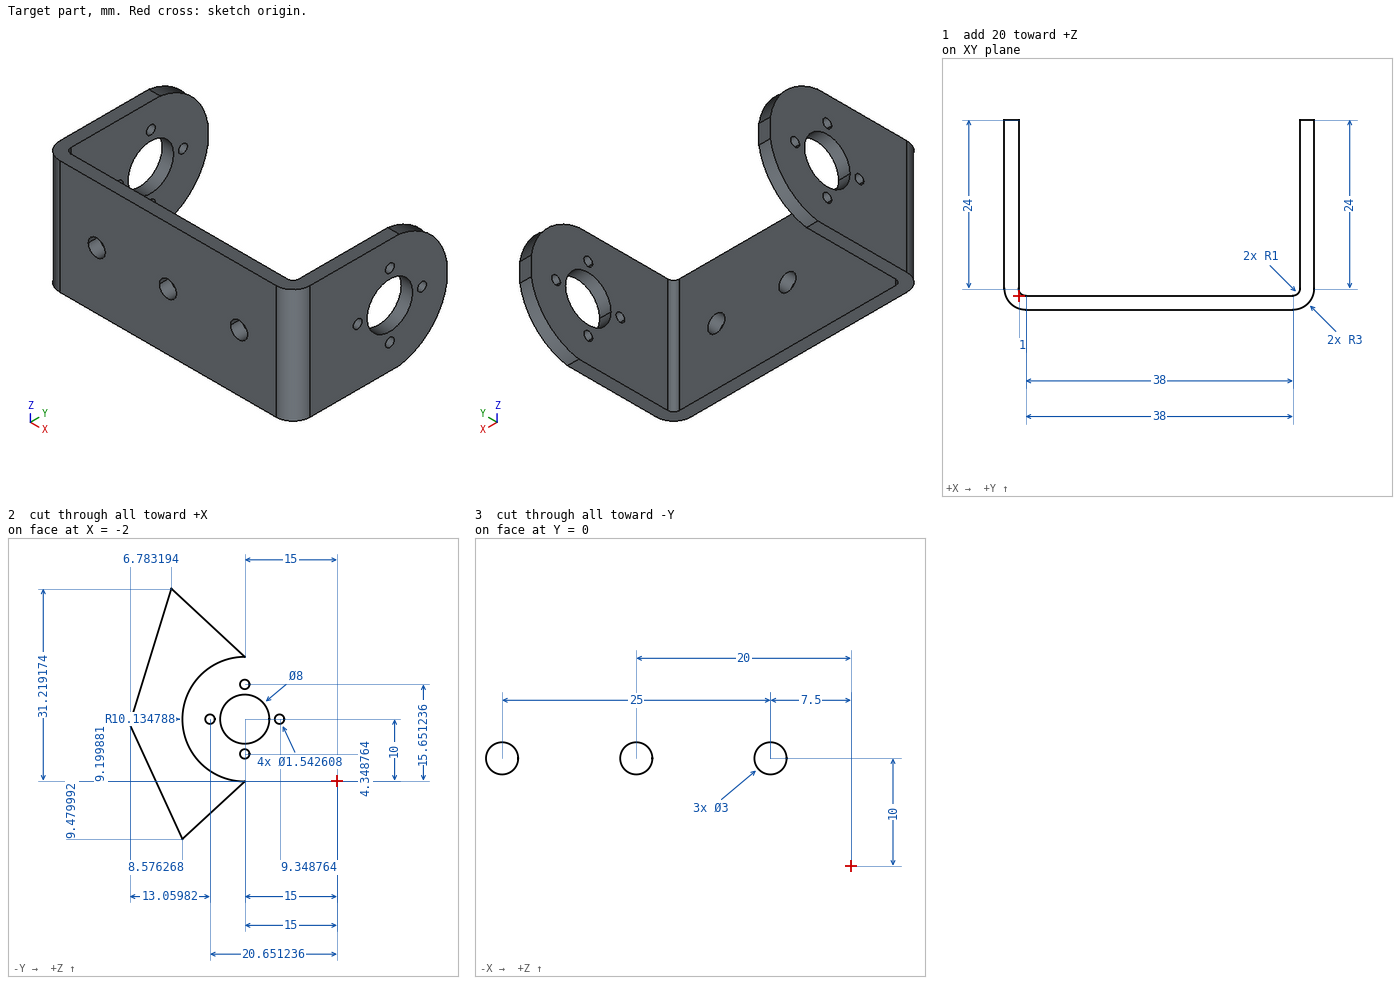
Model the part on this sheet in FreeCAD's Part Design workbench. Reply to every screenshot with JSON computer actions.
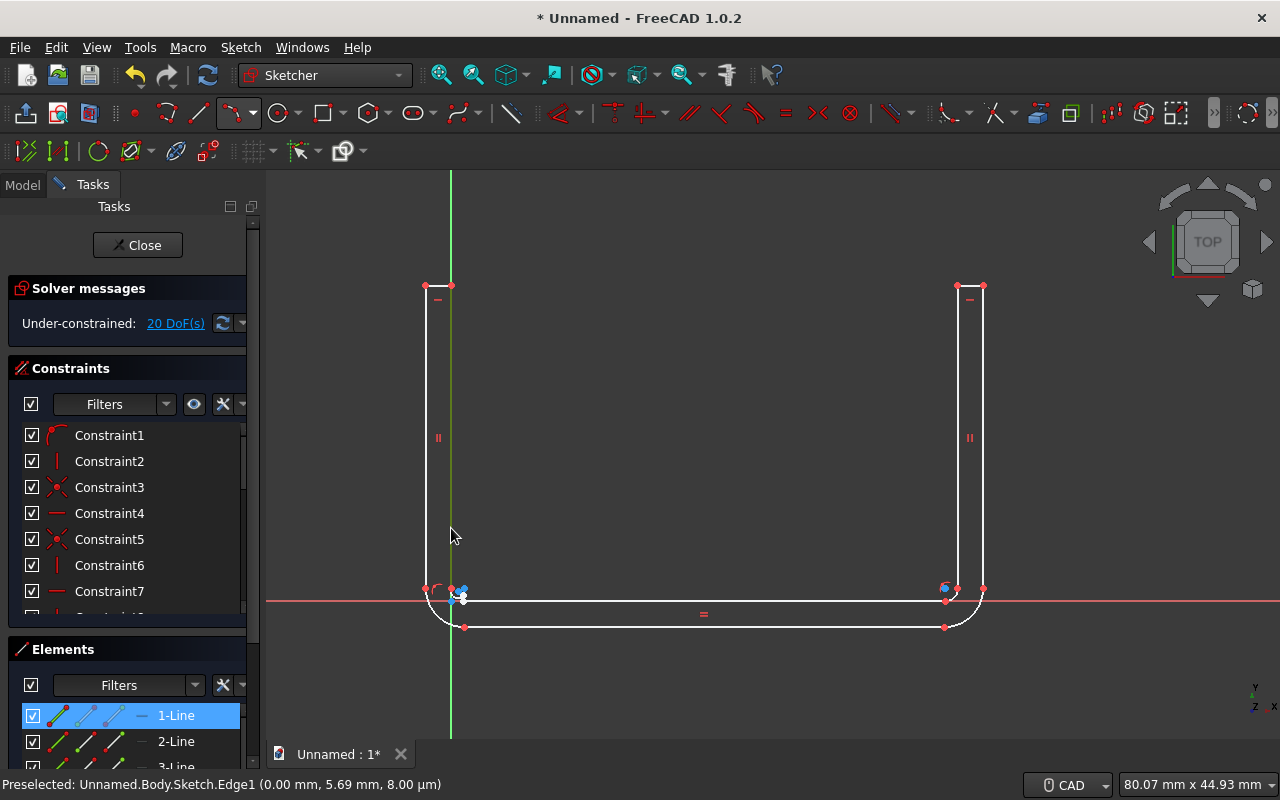
{"action": "scroll", "coordinate": [455, 597], "scroll_direction": "up", "scroll_amount": 4}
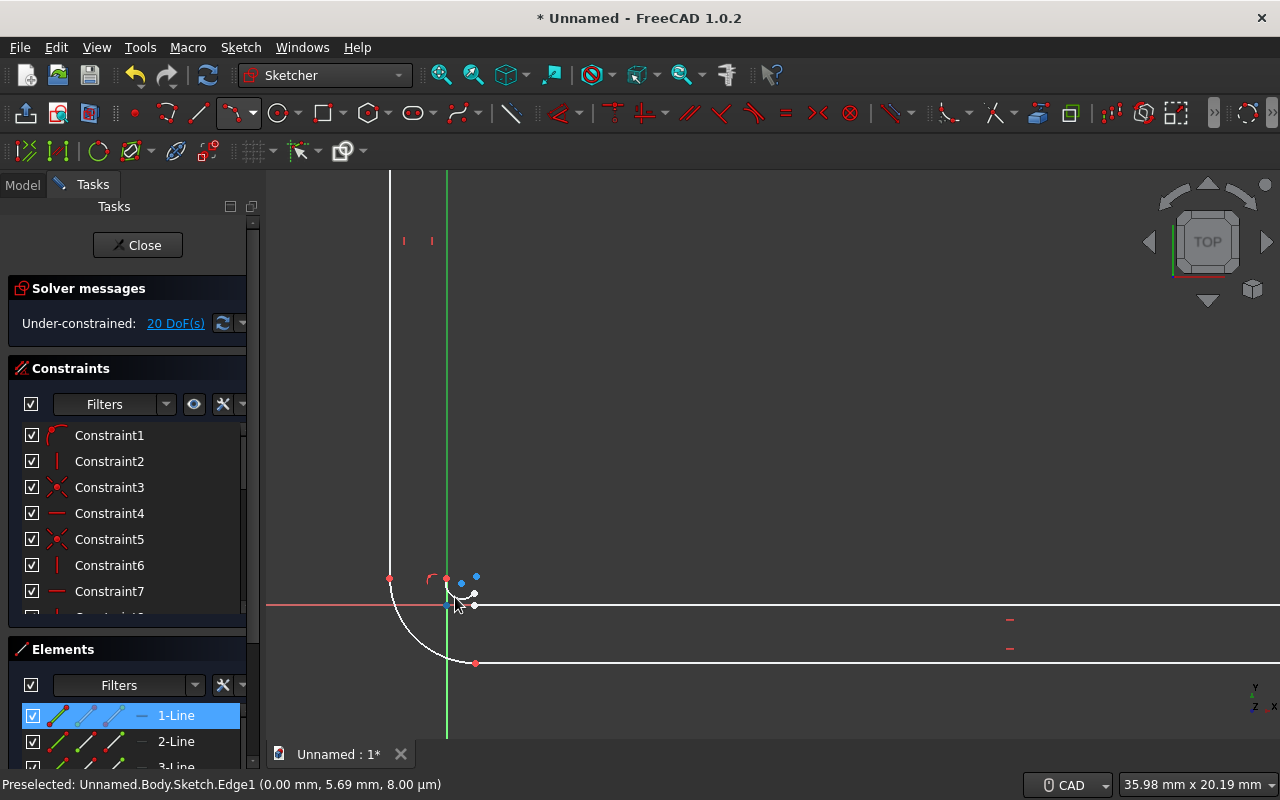
{"action": "left_click", "coordinate": [454, 597]}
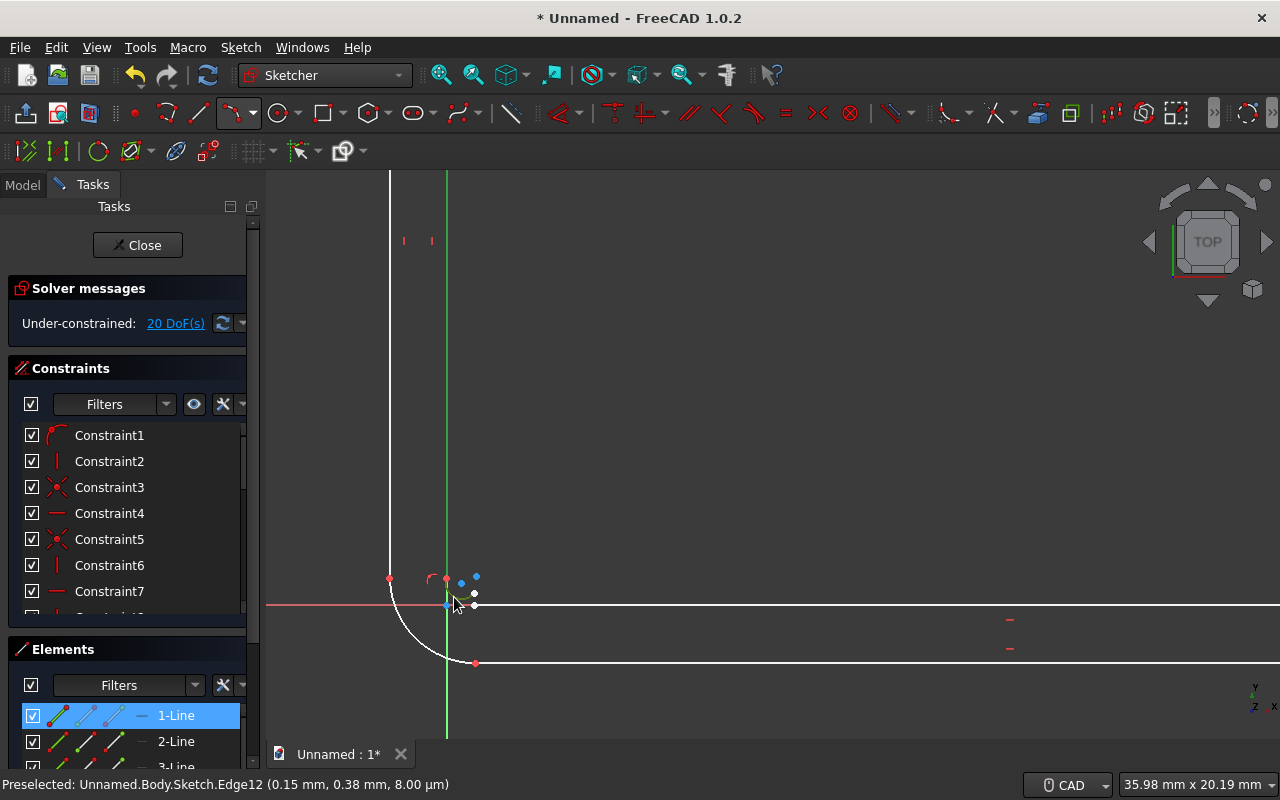
{"action": "left_click", "coordinate": [754, 114]}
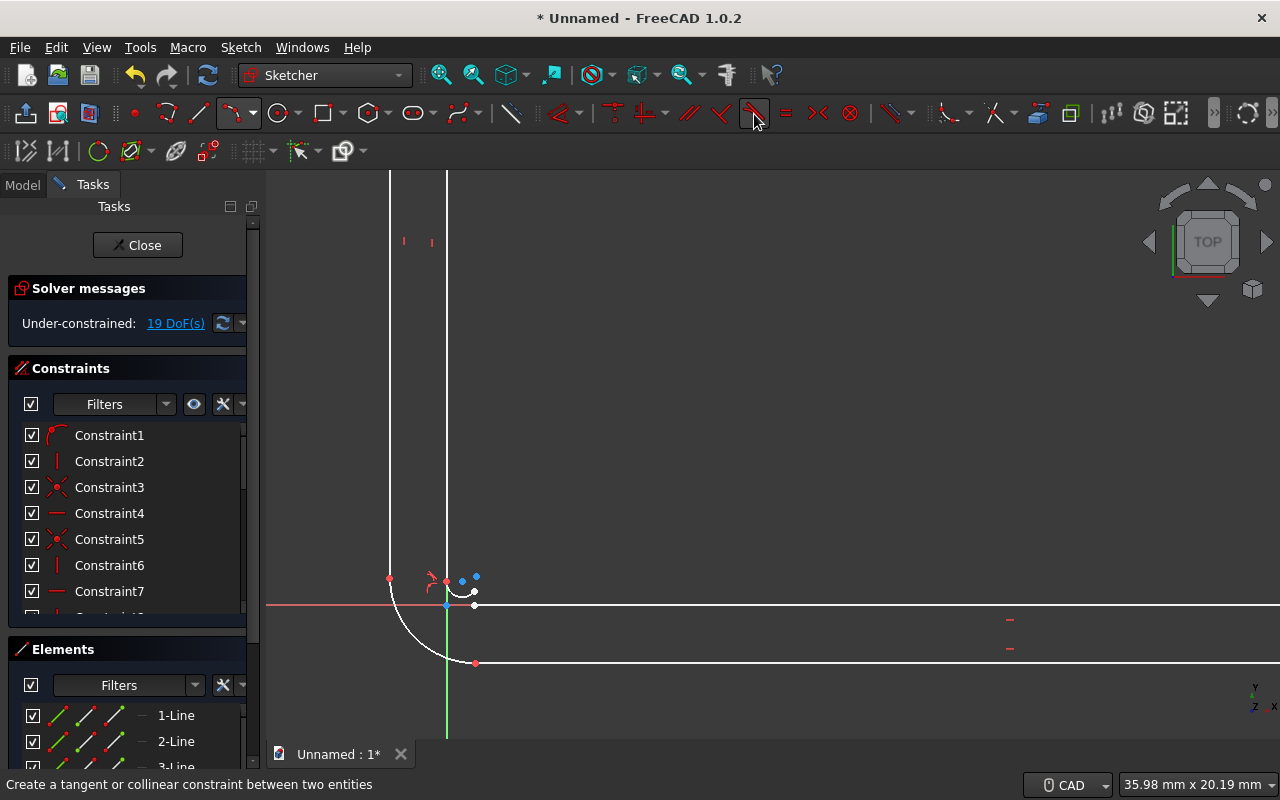
{"action": "left_click", "coordinate": [390, 376]}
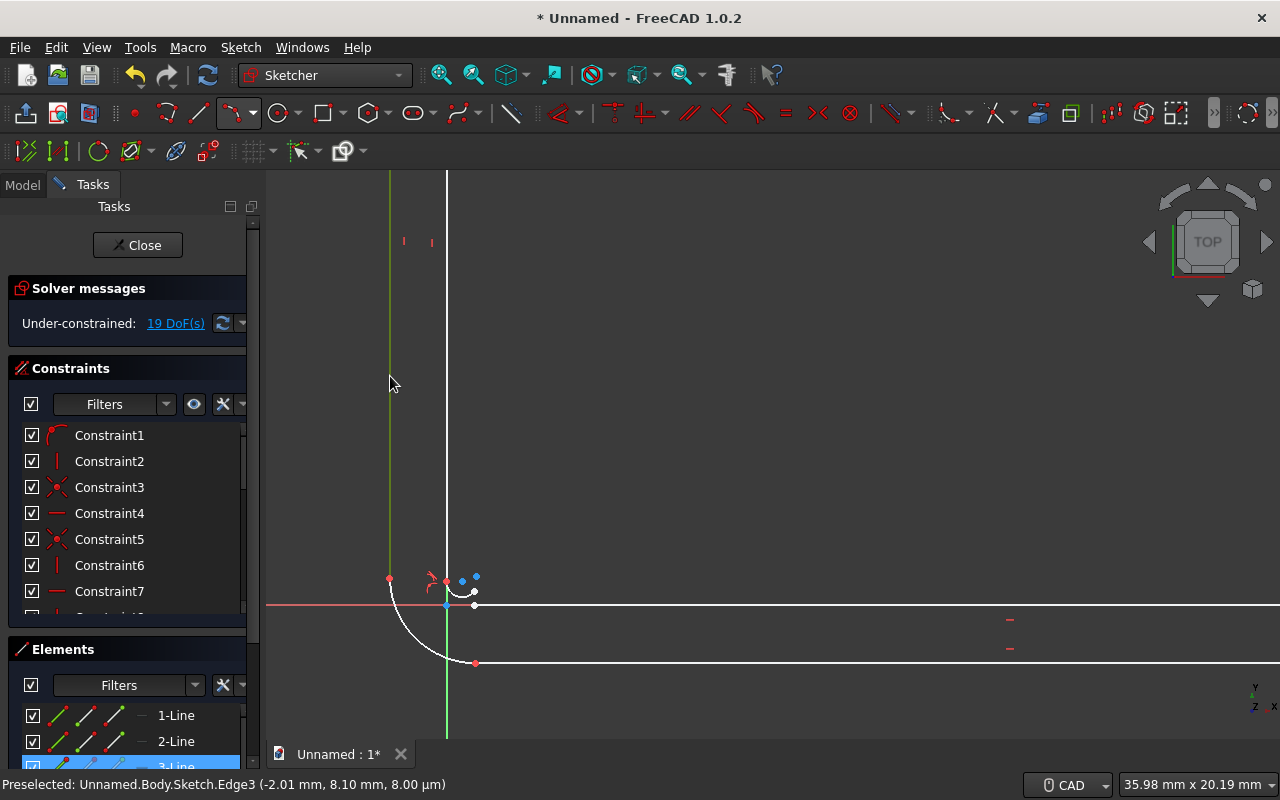
{"action": "left_click", "coordinate": [400, 617]}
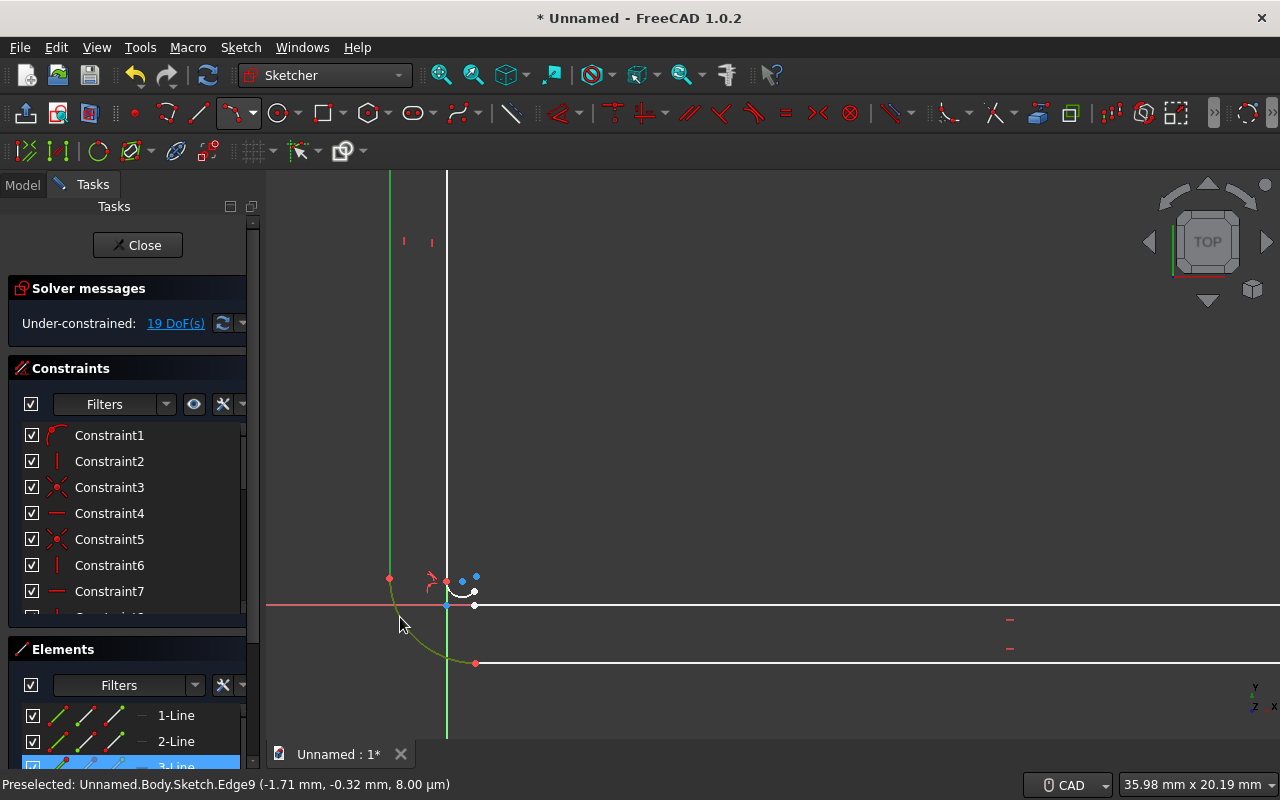
{"action": "key", "text": "t"}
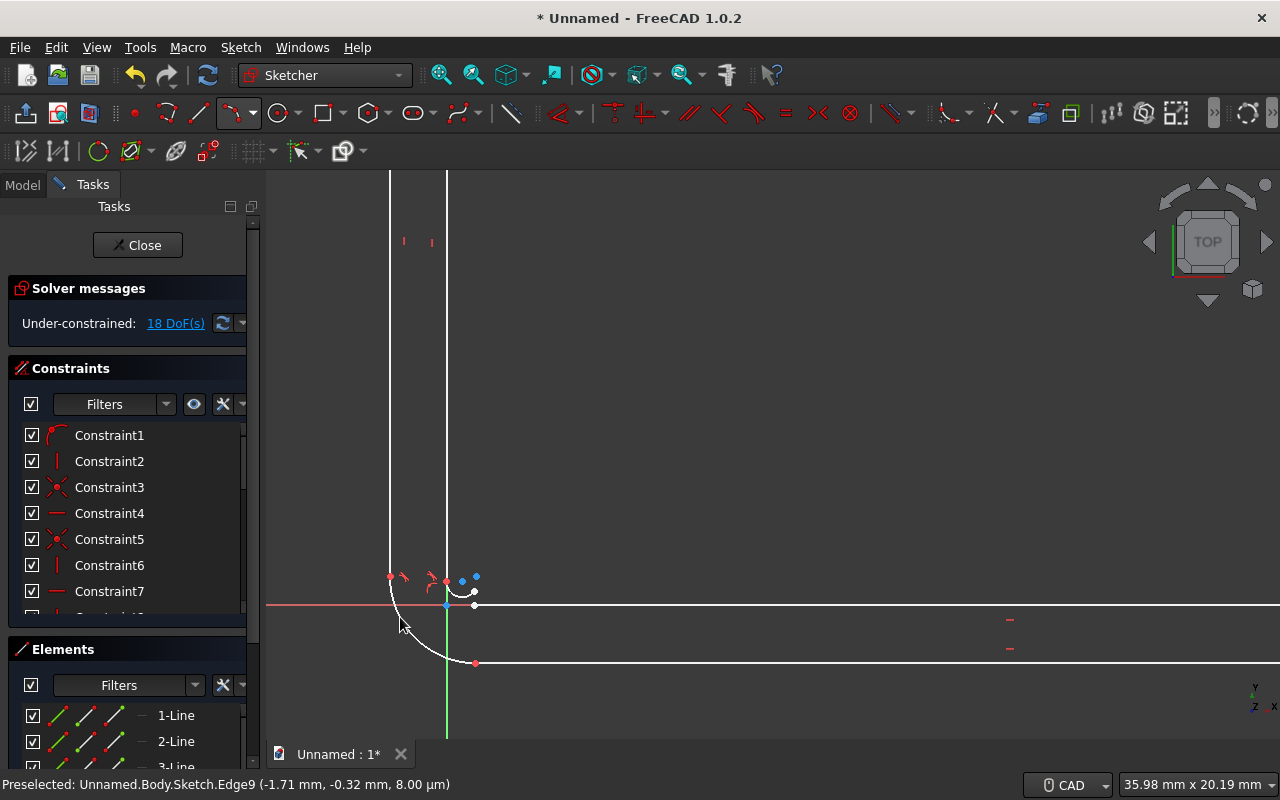
{"action": "left_click", "coordinate": [796, 663]}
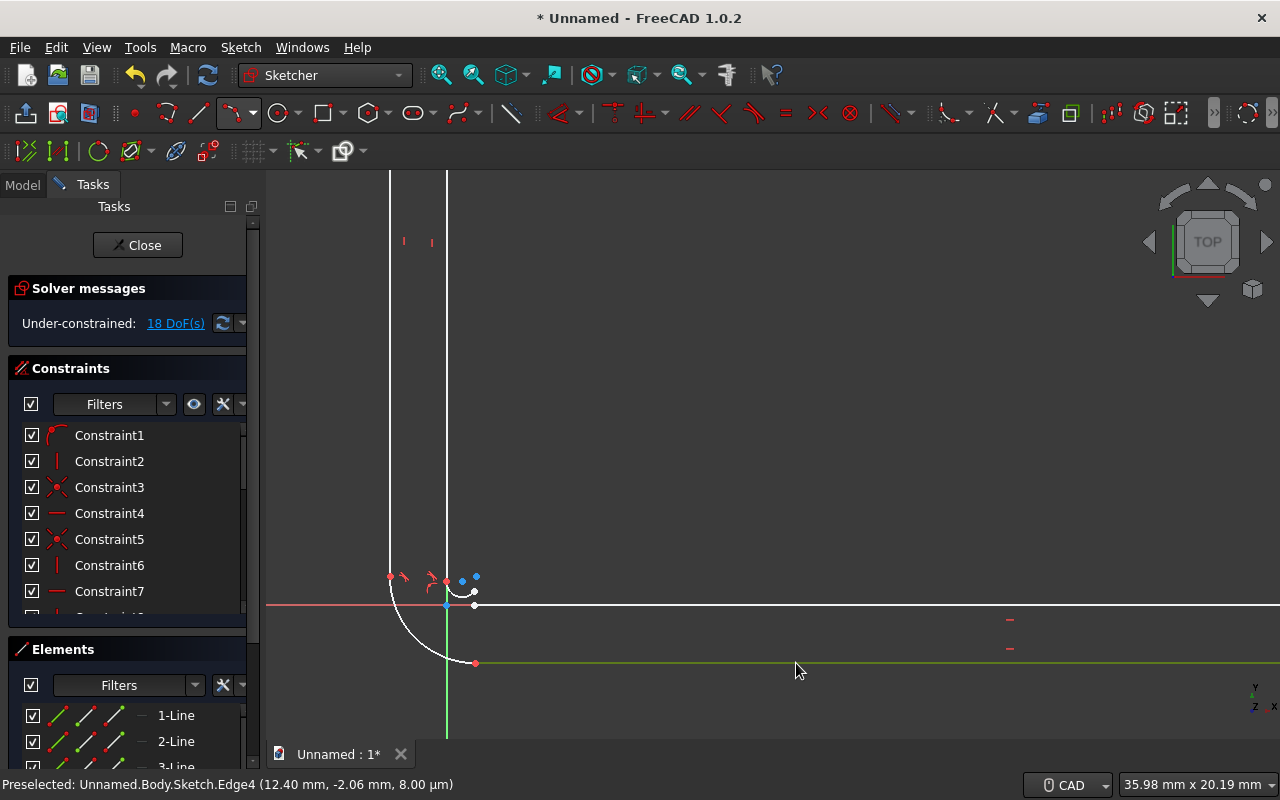
{"action": "scroll", "coordinate": [399, 616], "scroll_direction": "up", "scroll_amount": 2}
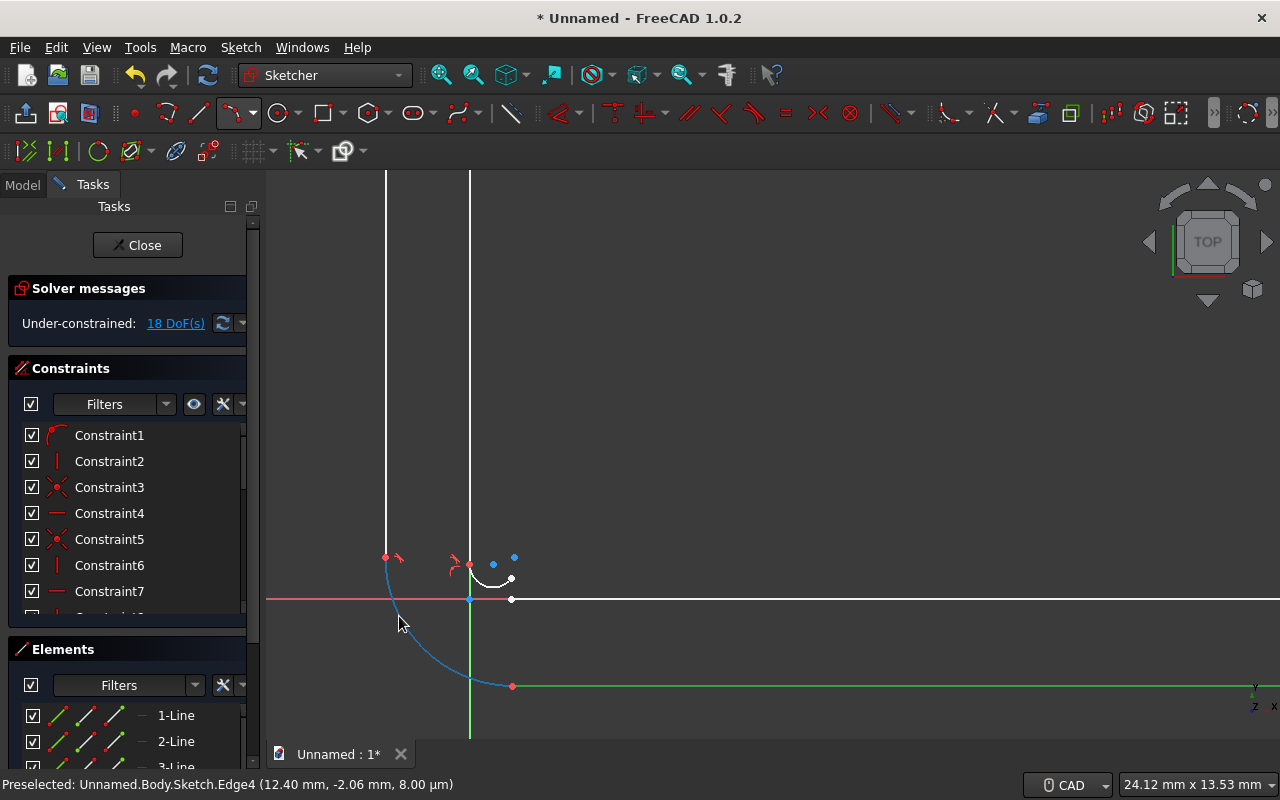
{"action": "left_click", "coordinate": [399, 615]}